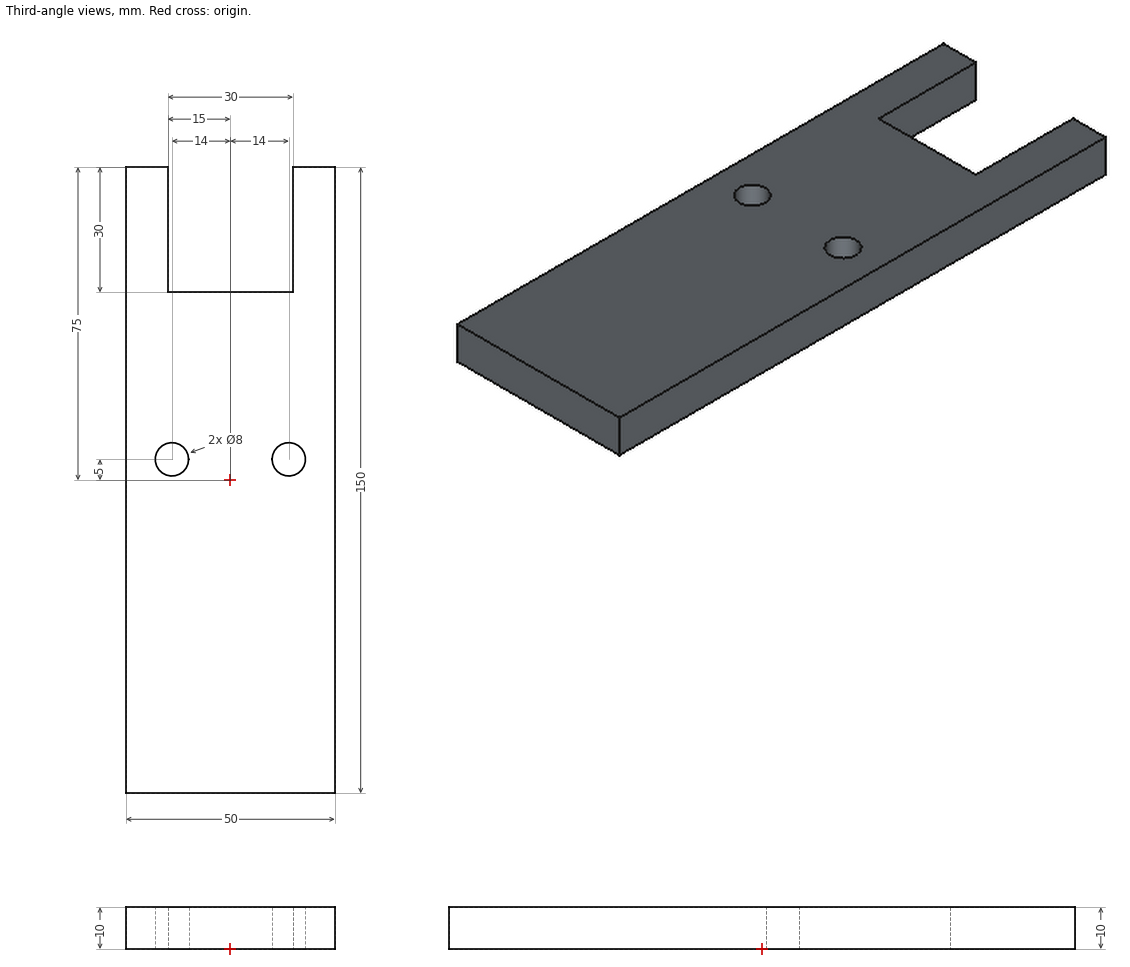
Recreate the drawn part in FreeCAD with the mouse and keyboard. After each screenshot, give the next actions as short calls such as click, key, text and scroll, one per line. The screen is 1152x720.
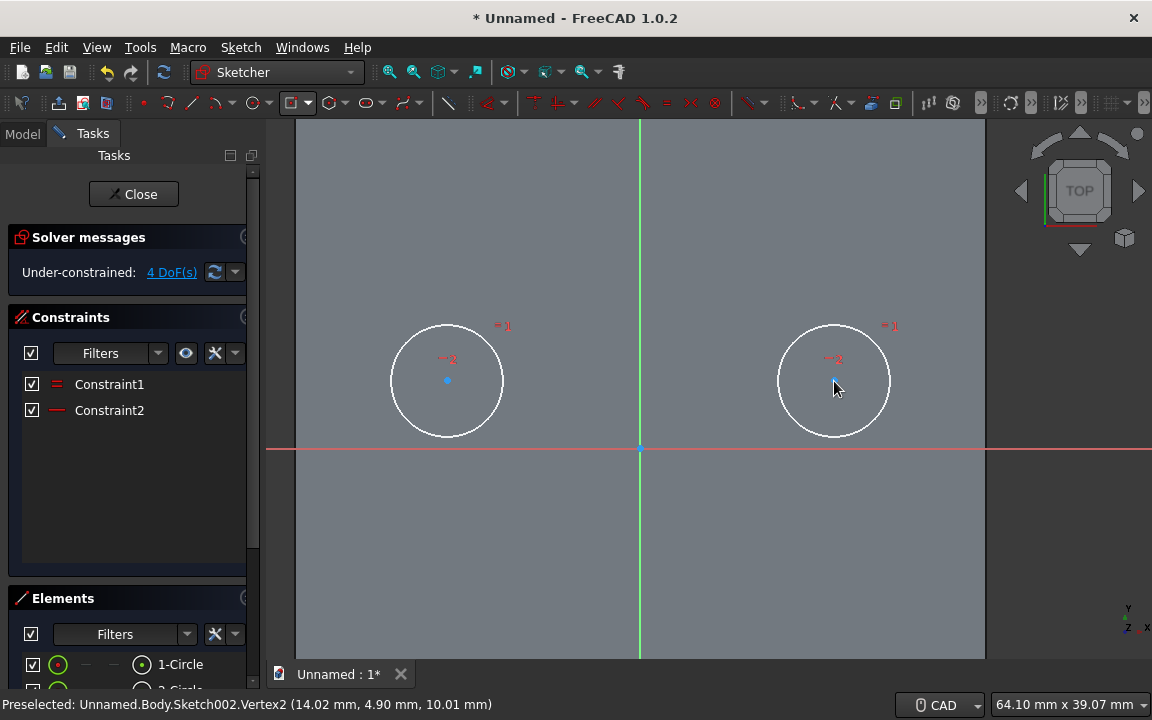
click(488, 104)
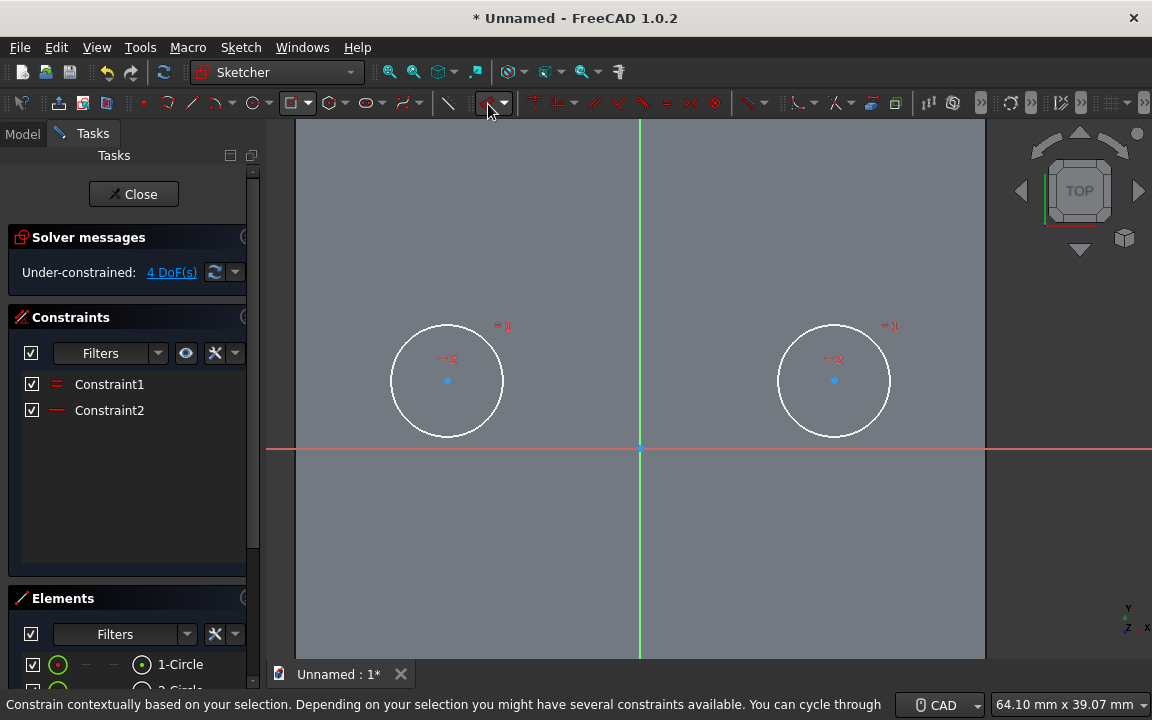
click(486, 341)
click(508, 318)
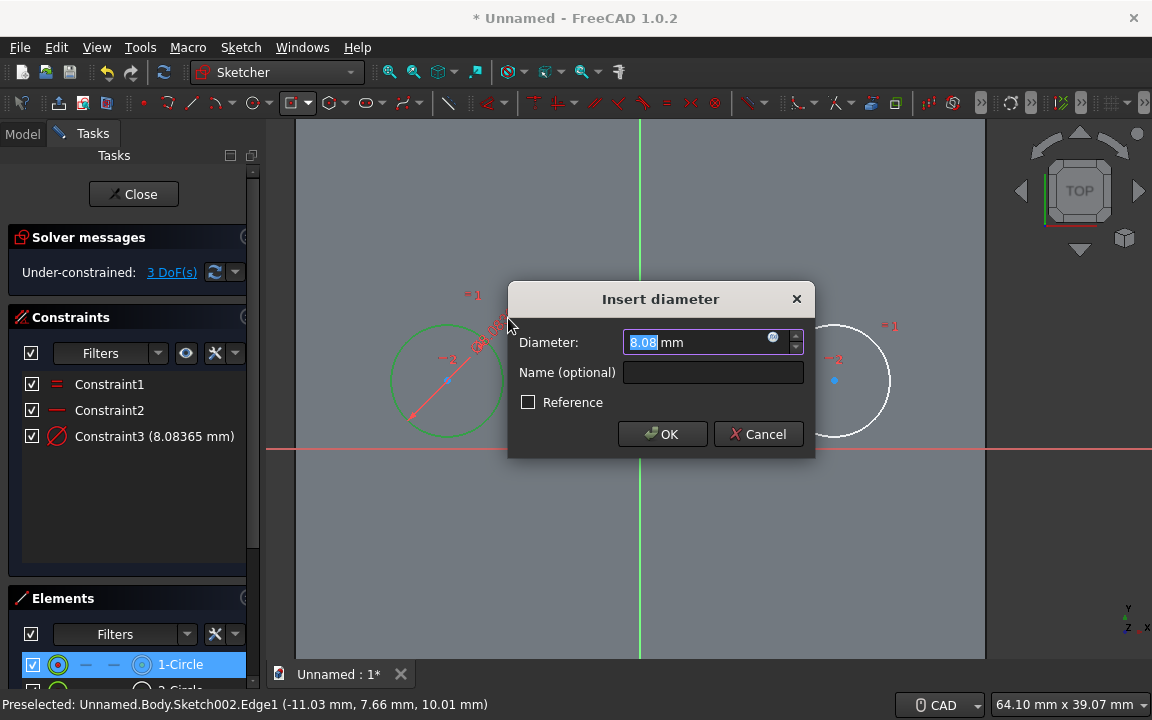
text(8)
key(Return)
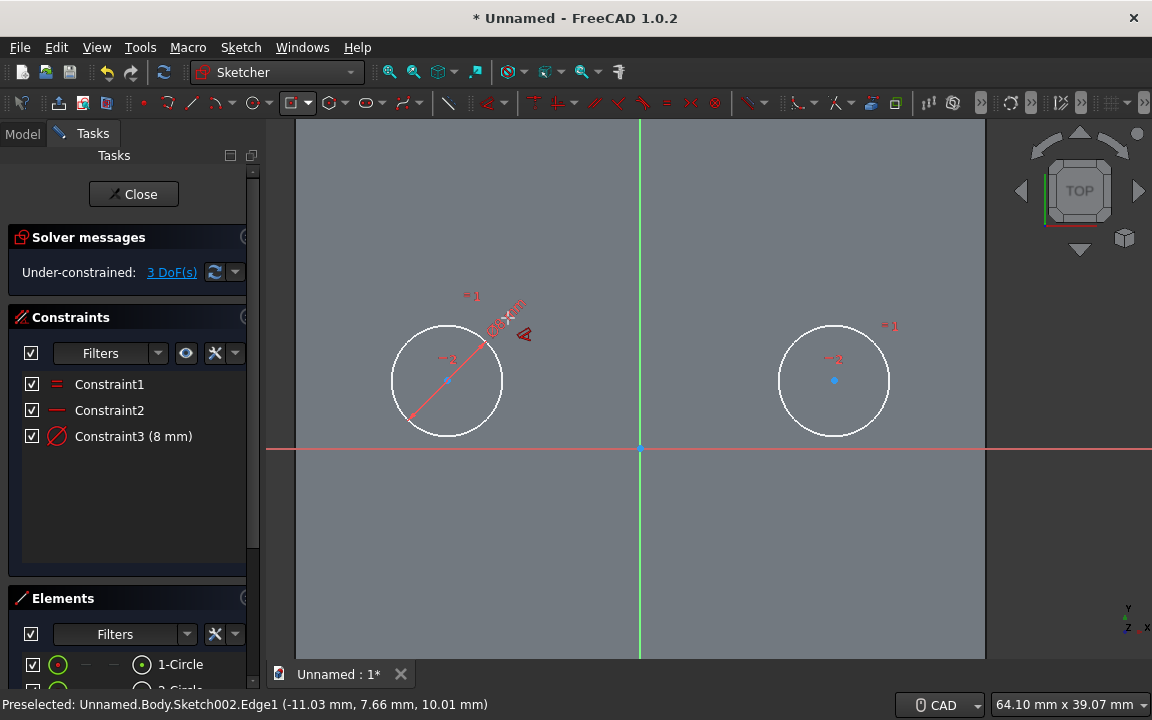
click(447, 381)
click(413, 399)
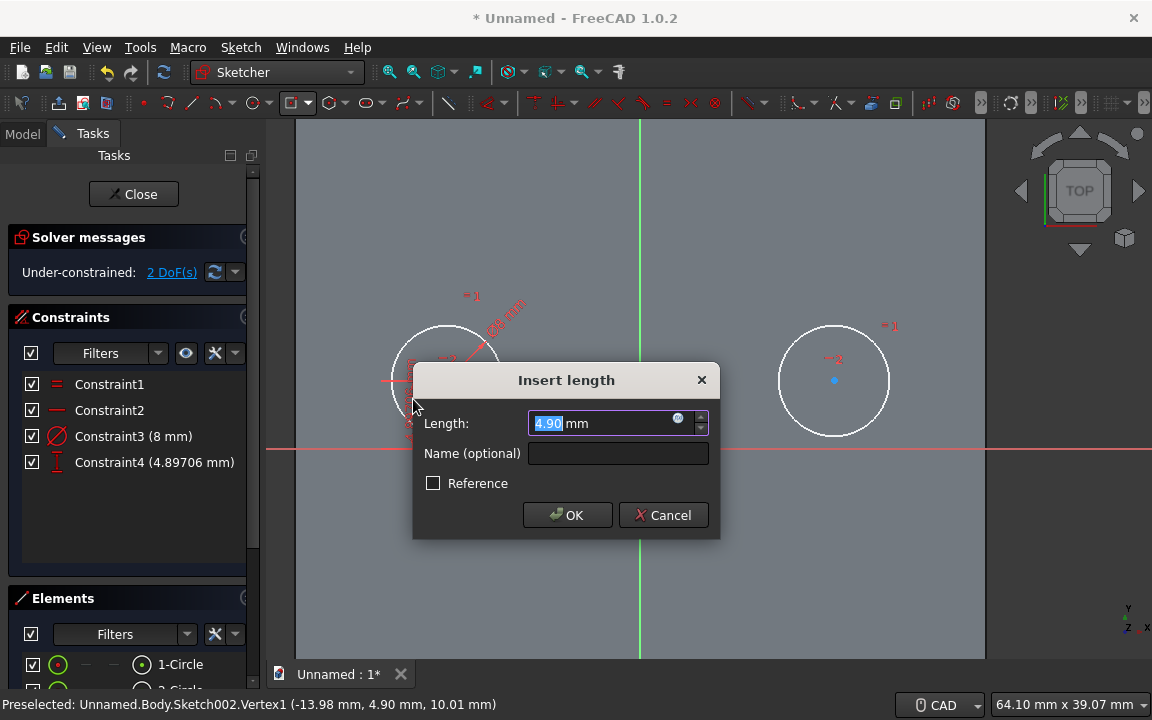
text(5)
key(Return)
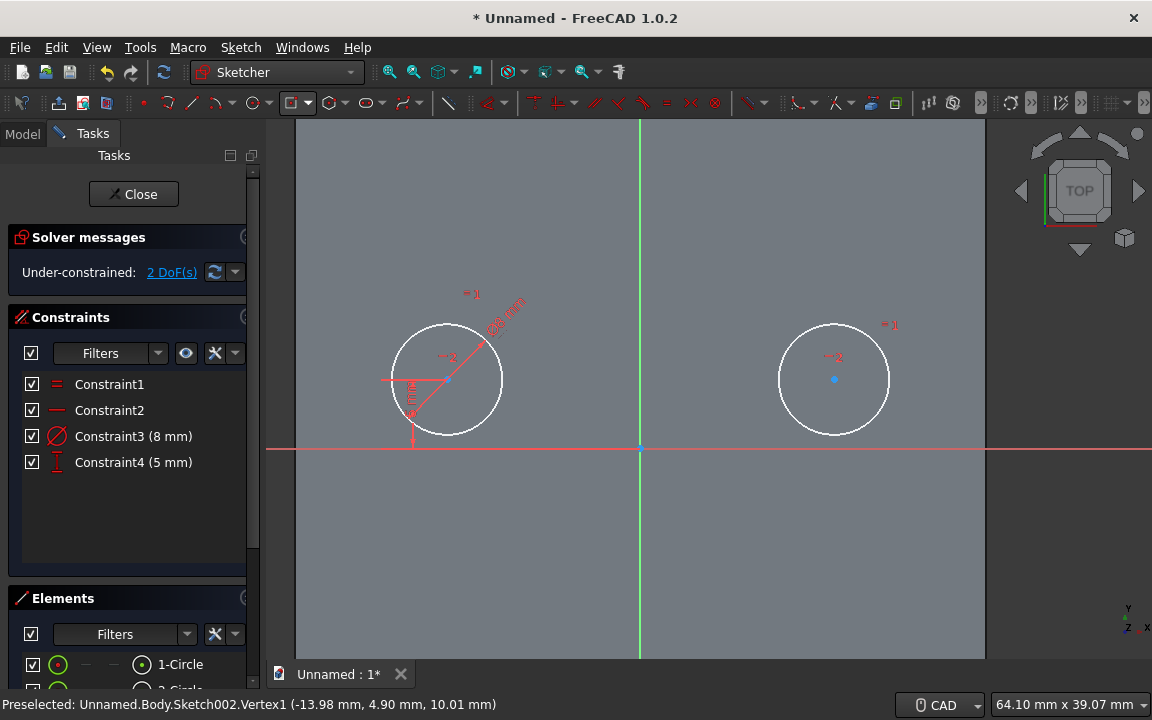
click(447, 380)
click(544, 483)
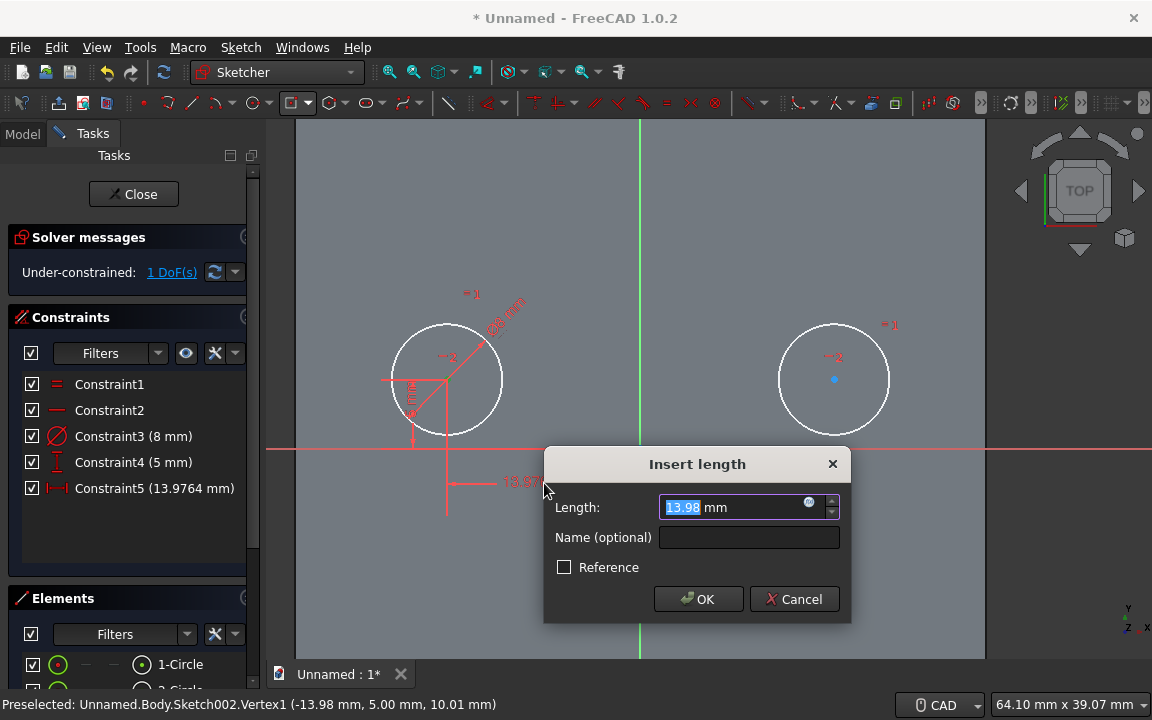
text(14)
key(Return)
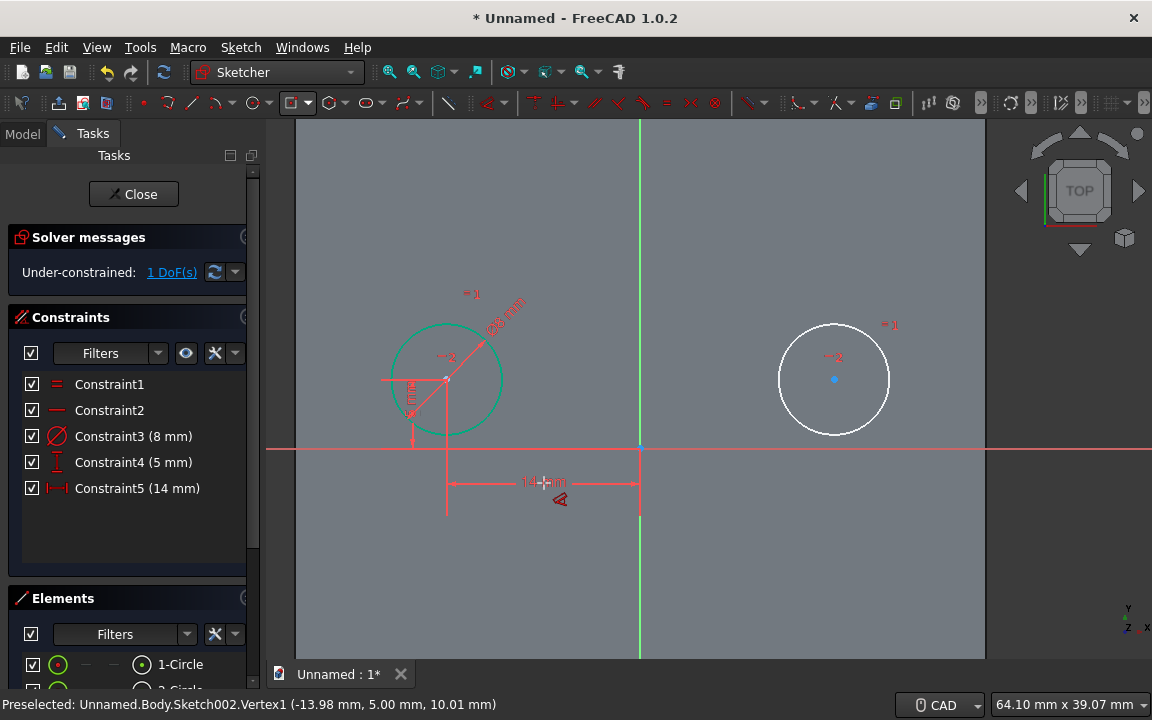
click(834, 380)
click(737, 483)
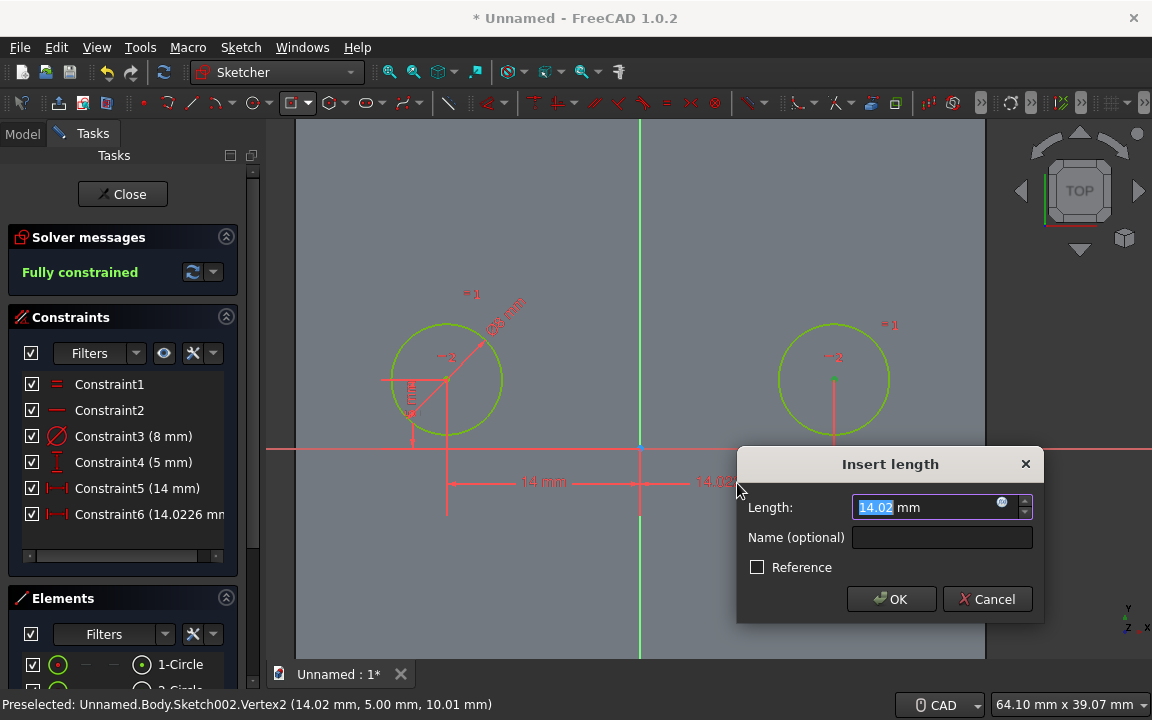
text(14)
key(Return)
key(Escape)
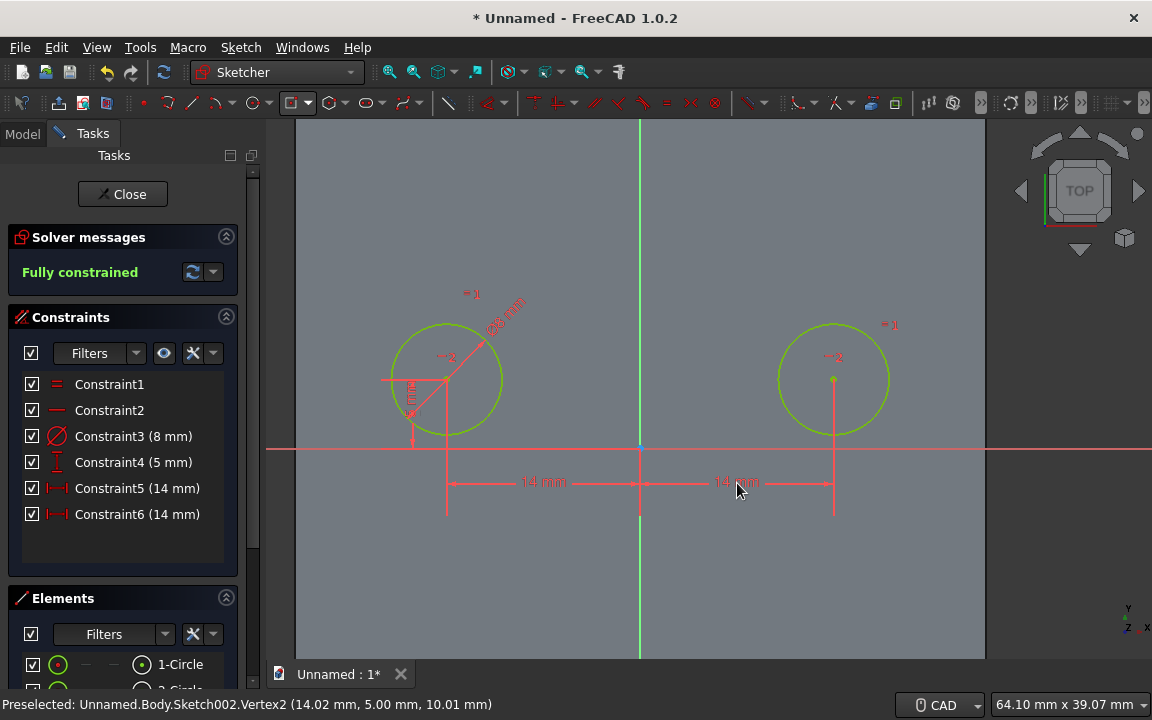
click(123, 194)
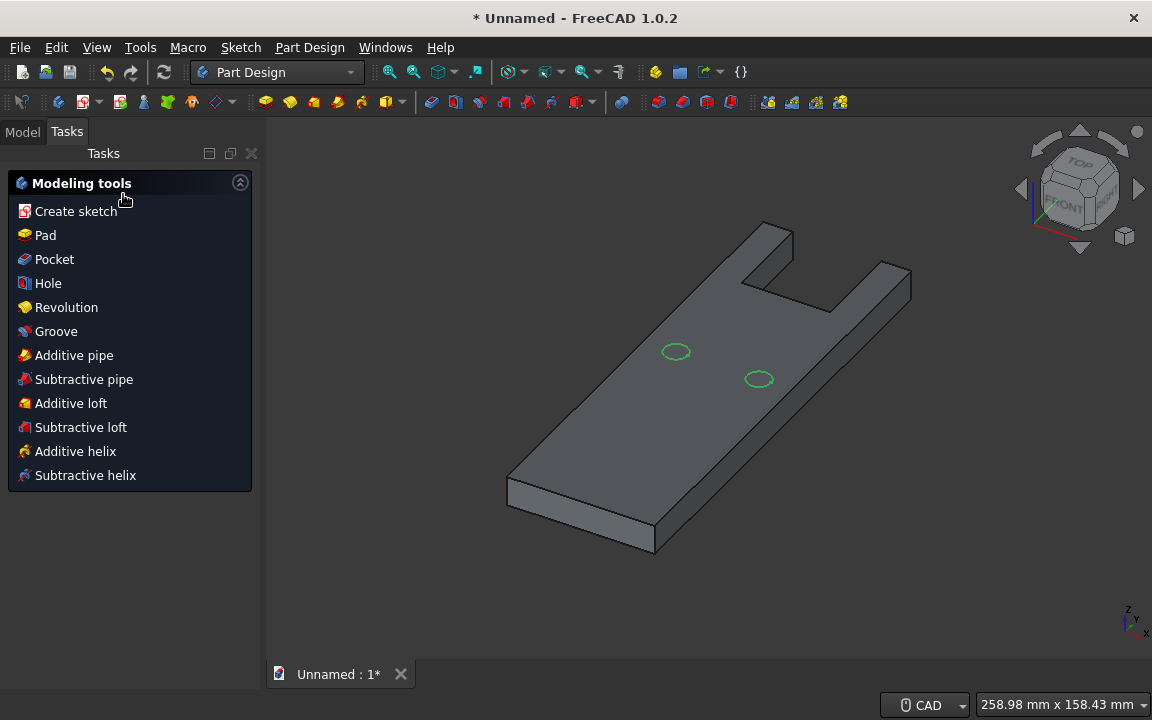
click(432, 102)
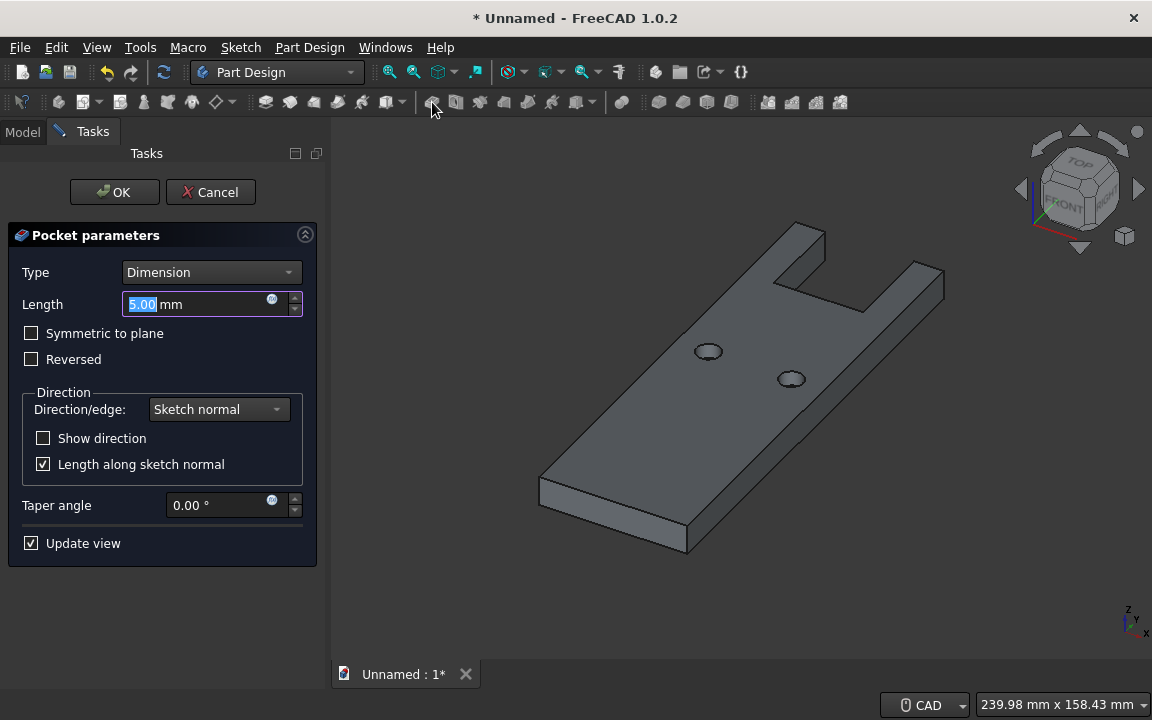
click(212, 272)